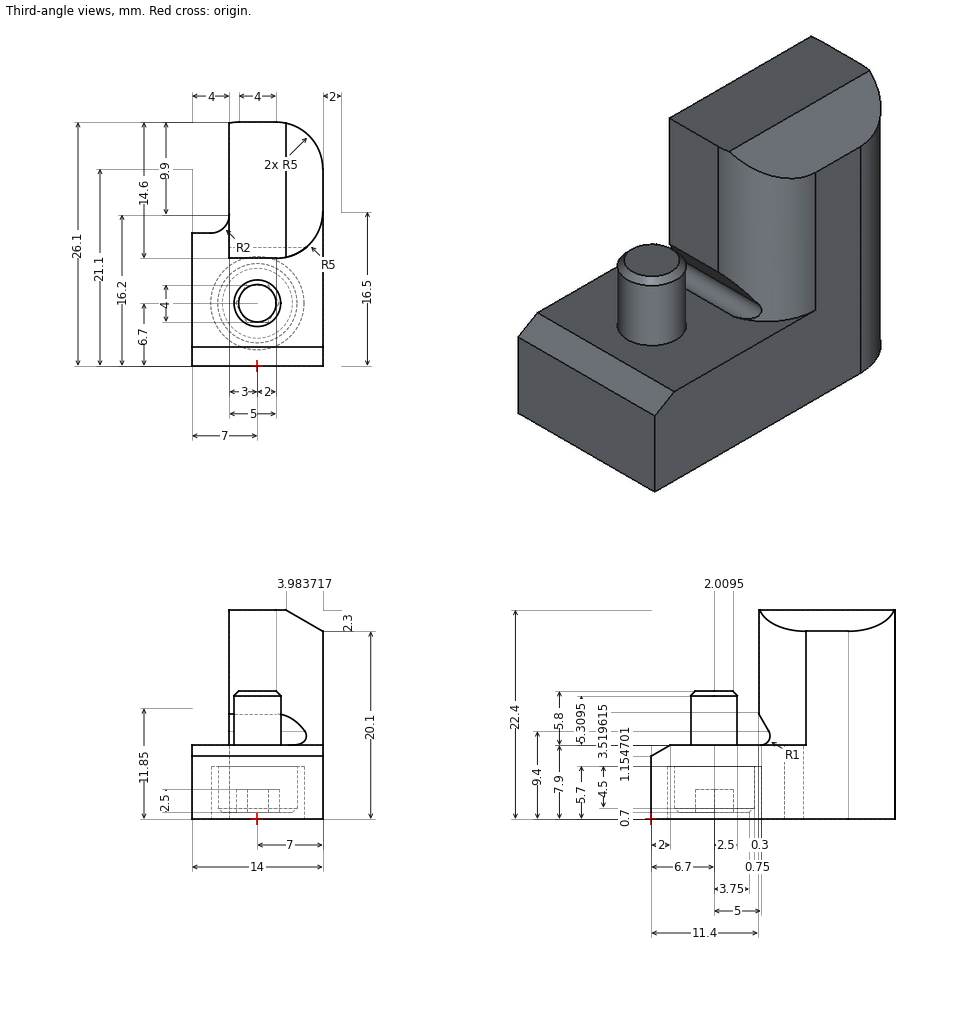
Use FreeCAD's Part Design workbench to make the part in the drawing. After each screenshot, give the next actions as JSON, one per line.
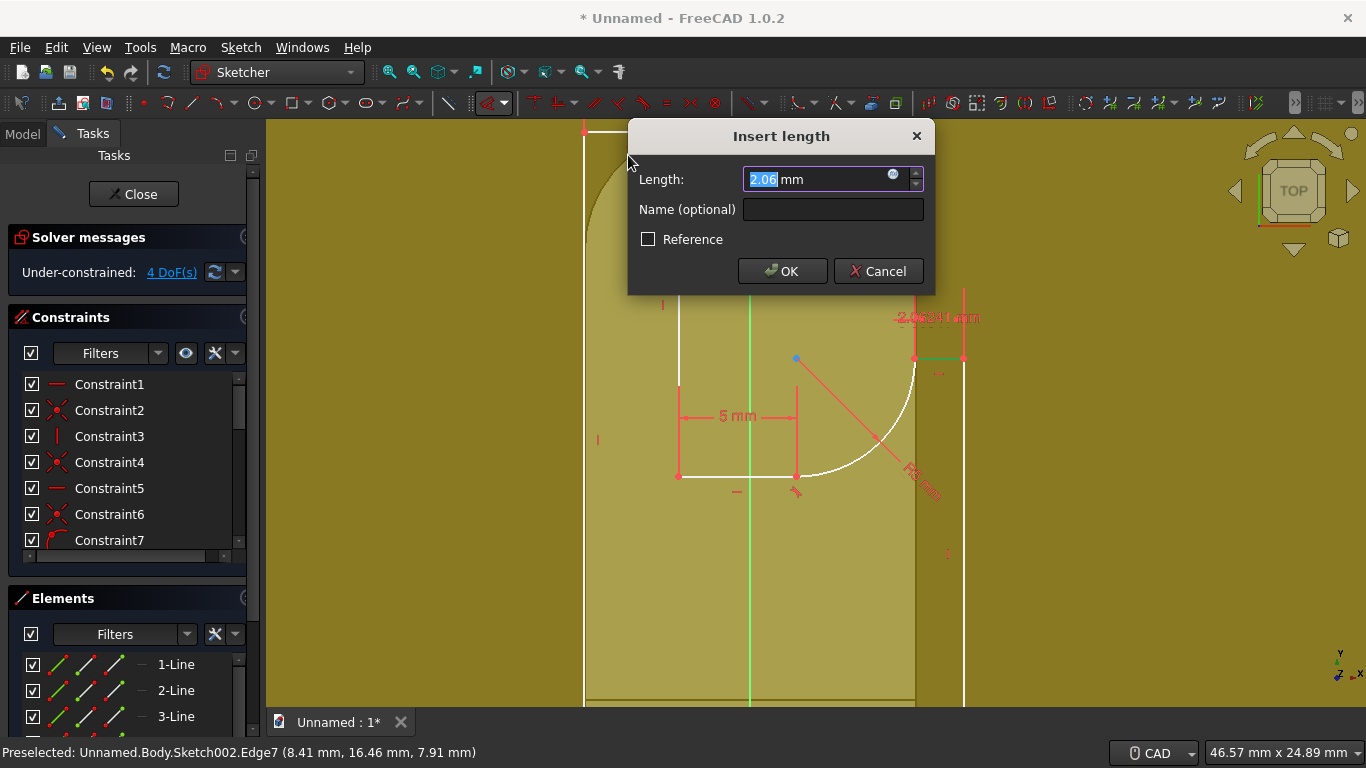
{"action": "type", "text": "2"}
{"action": "key", "text": "Return"}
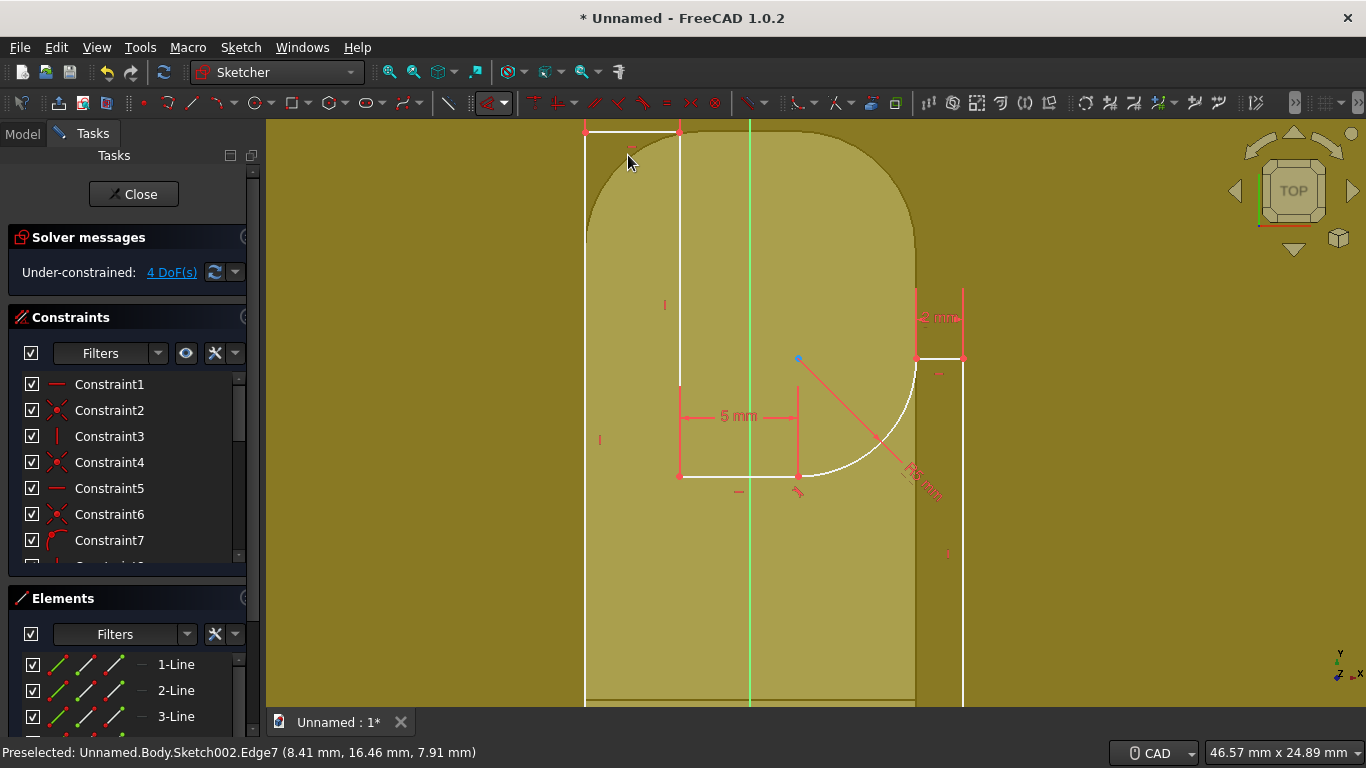
{"action": "left_click", "coordinate": [798, 477]}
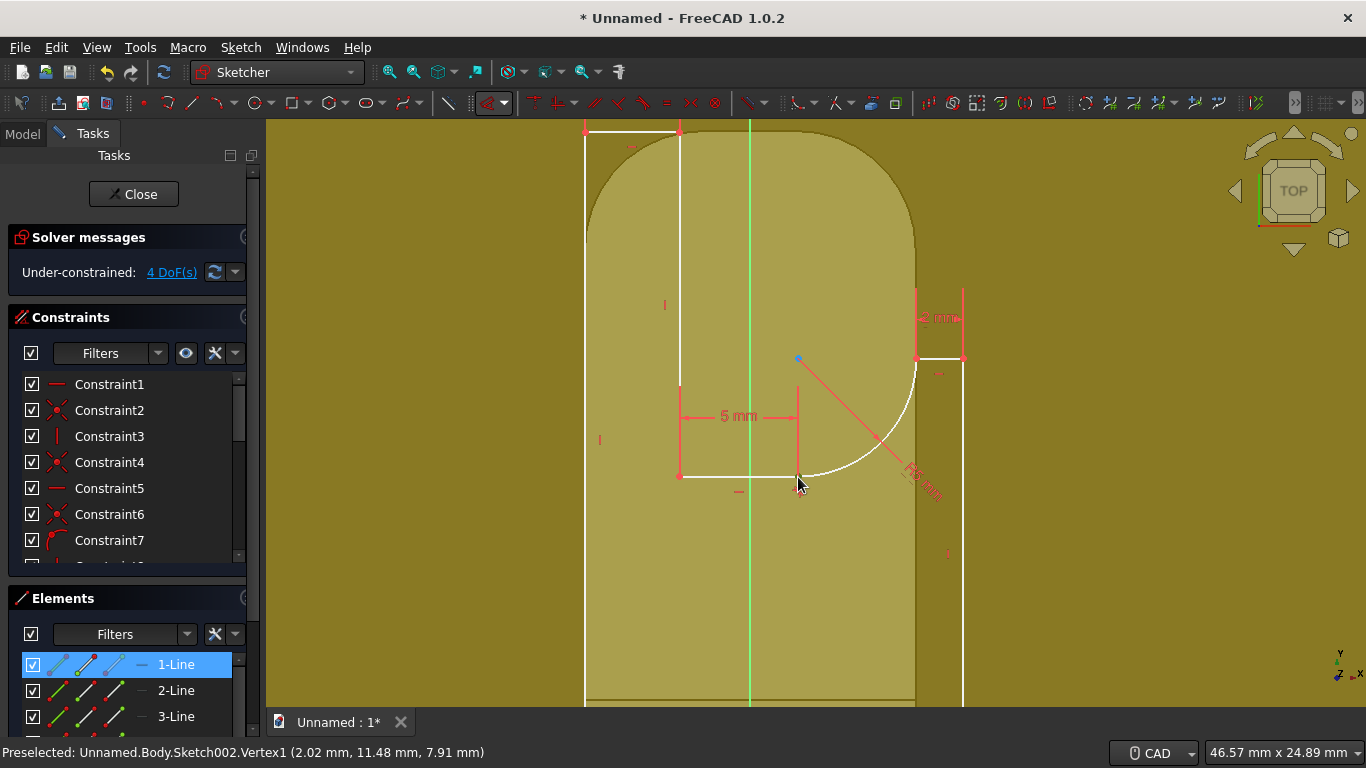
{"action": "key", "text": "l"}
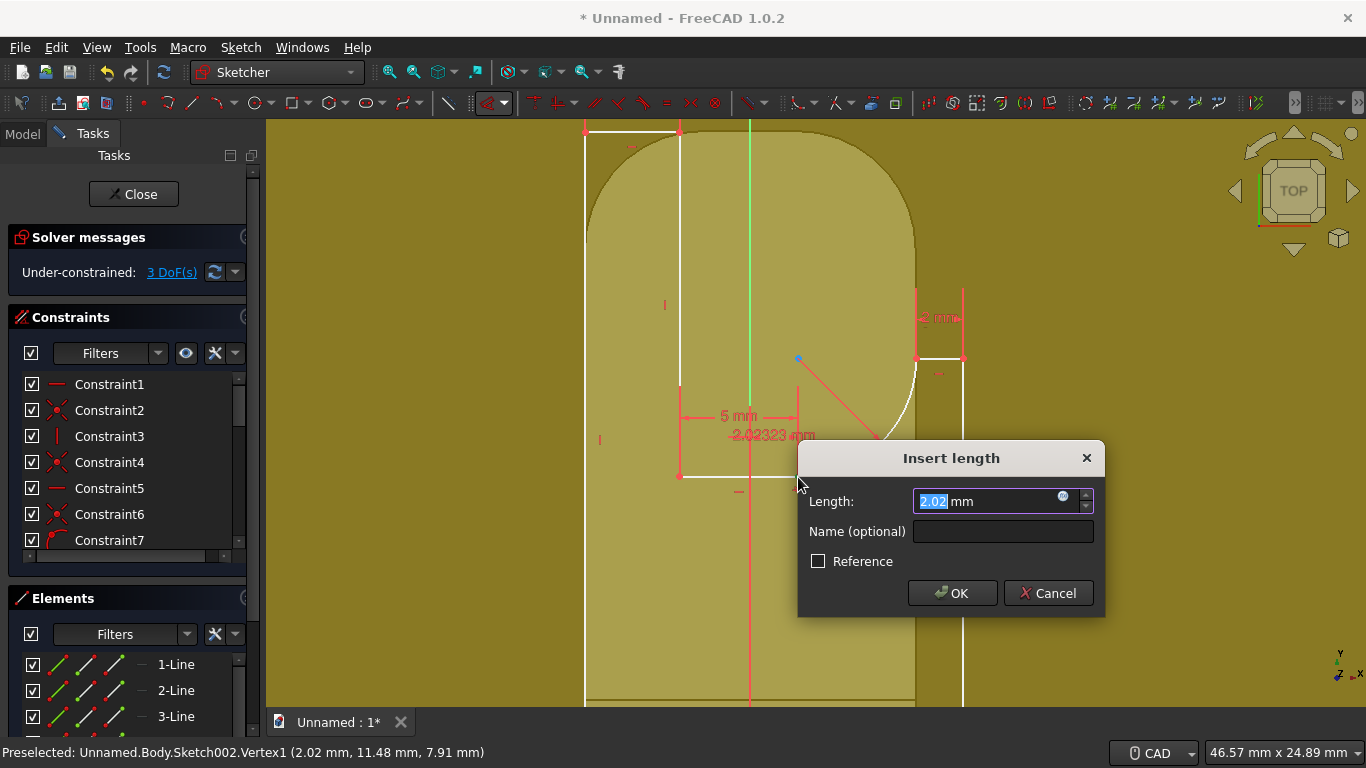
{"action": "type", "text": "2"}
{"action": "key", "text": "Return"}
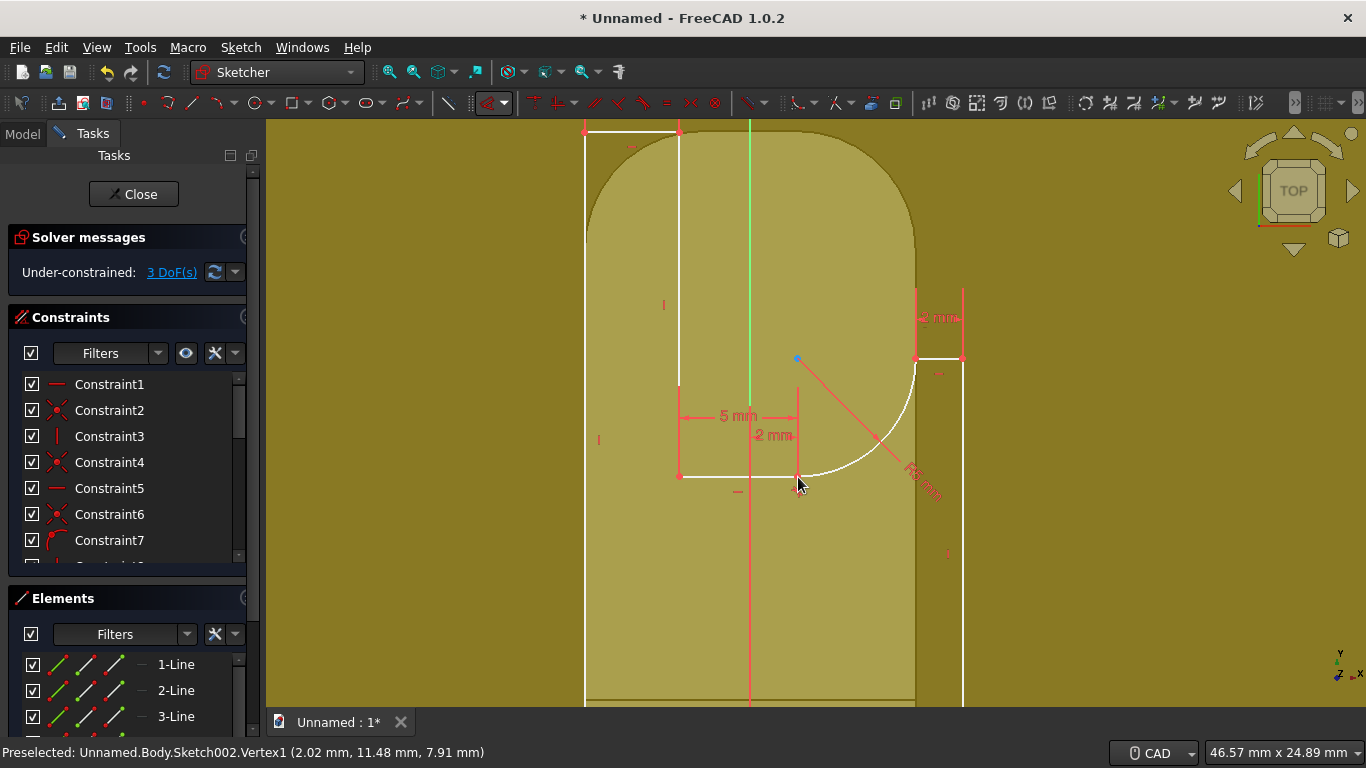
{"action": "left_click", "coordinate": [679, 373]}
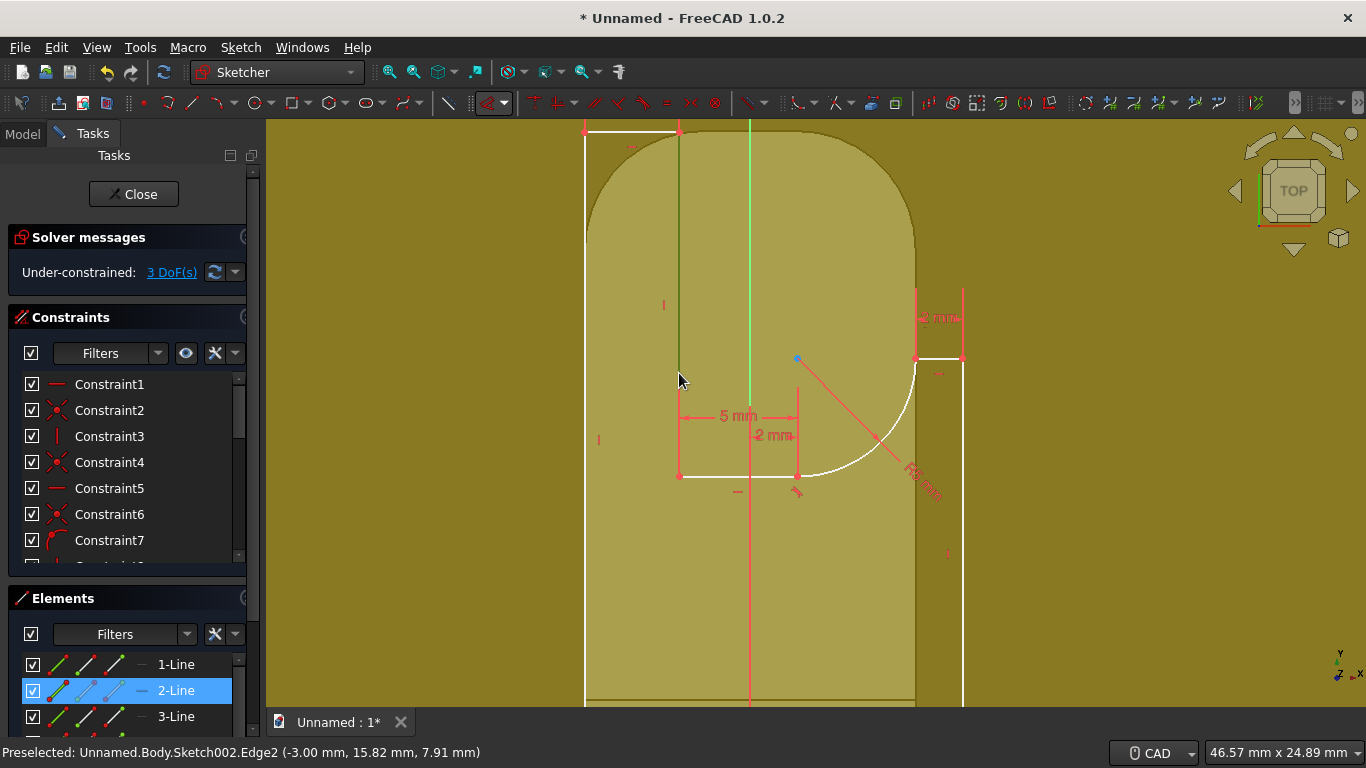
{"action": "left_click", "coordinate": [506, 104]}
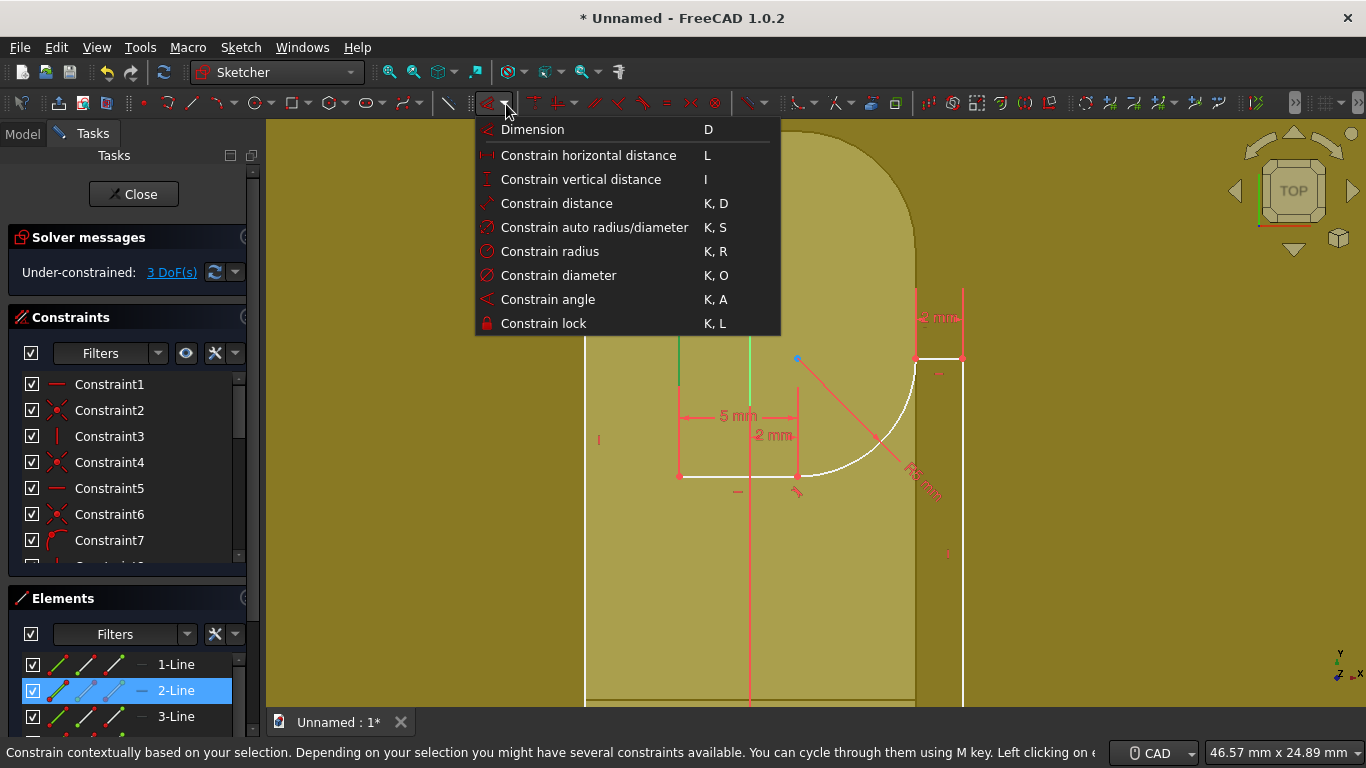
{"action": "left_click", "coordinate": [628, 179]}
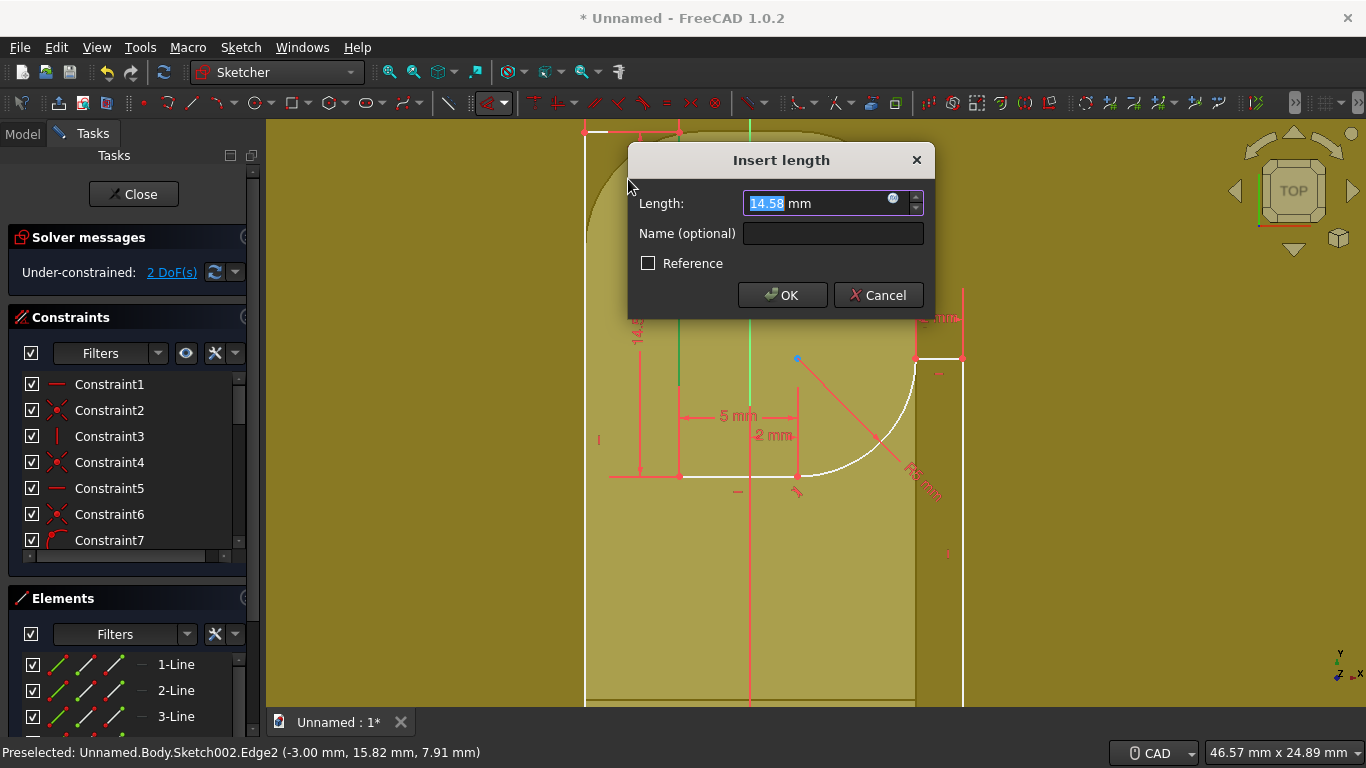
{"action": "type", "text": "14.6"}
{"action": "key", "text": "Return"}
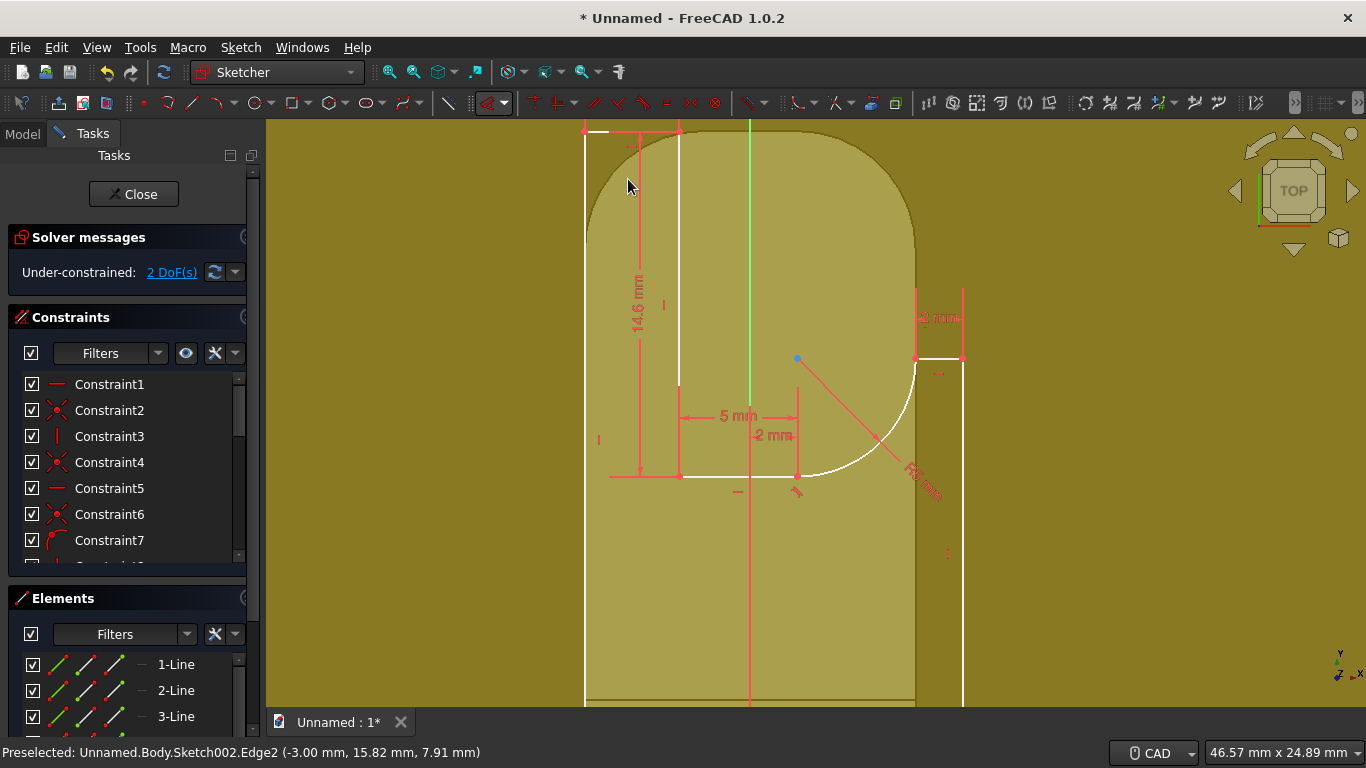
{"action": "left_click", "coordinate": [585, 316]}